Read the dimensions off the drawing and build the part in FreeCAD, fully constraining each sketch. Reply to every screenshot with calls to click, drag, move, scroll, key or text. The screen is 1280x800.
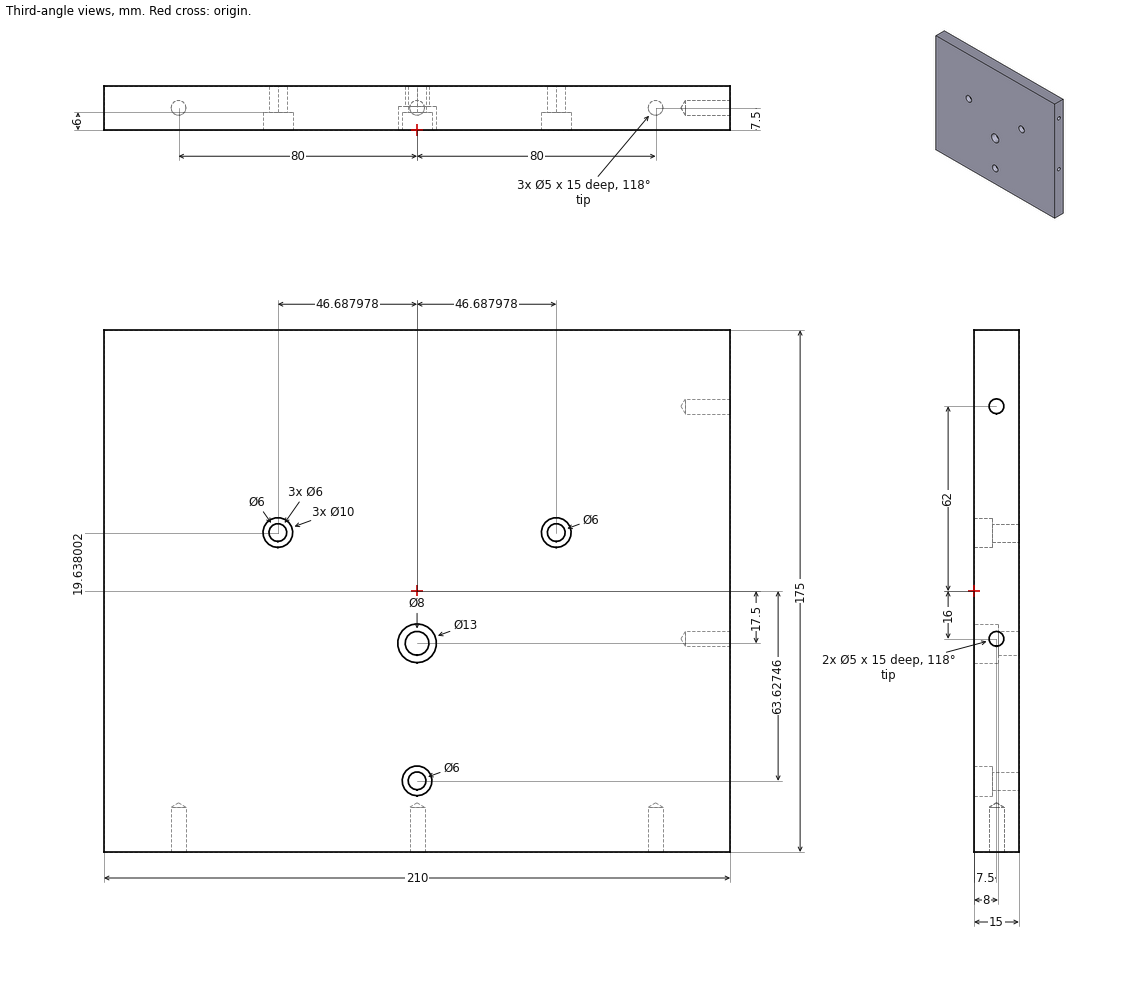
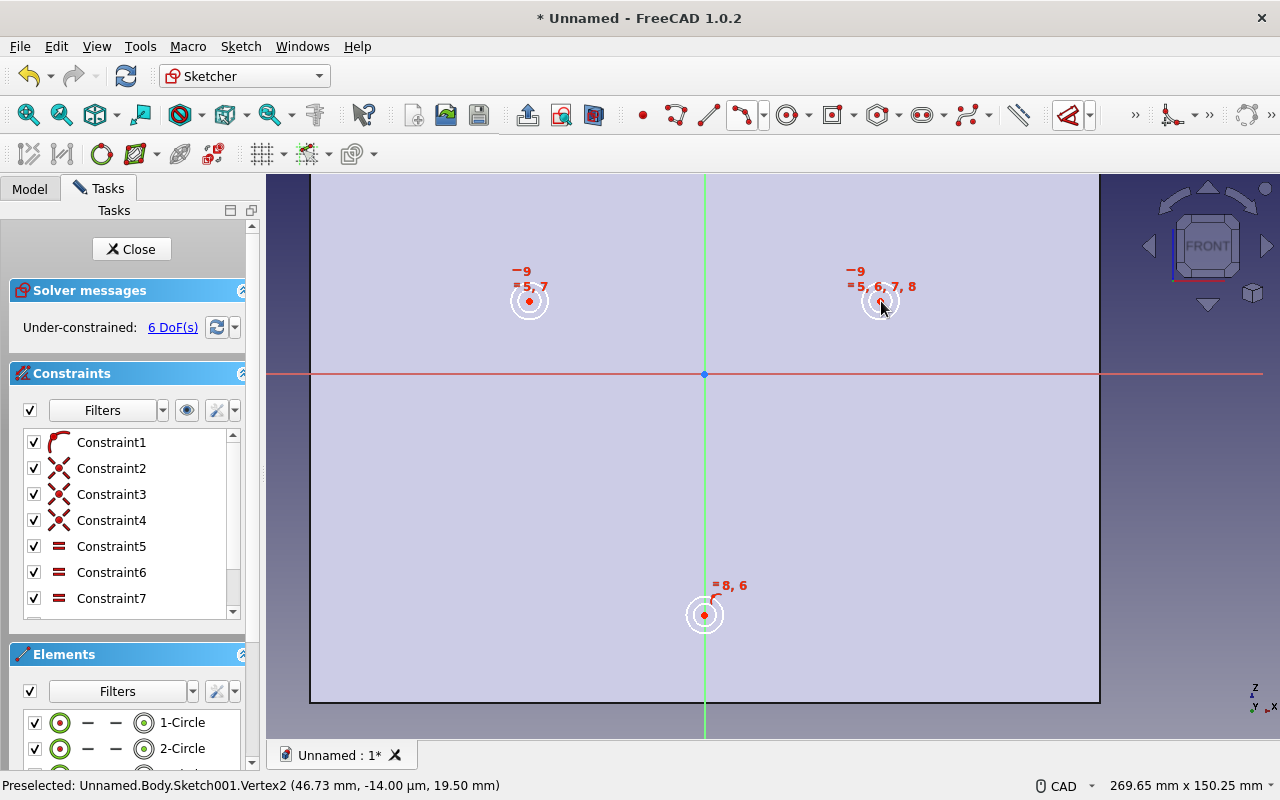
scroll(543, 288, up, 4)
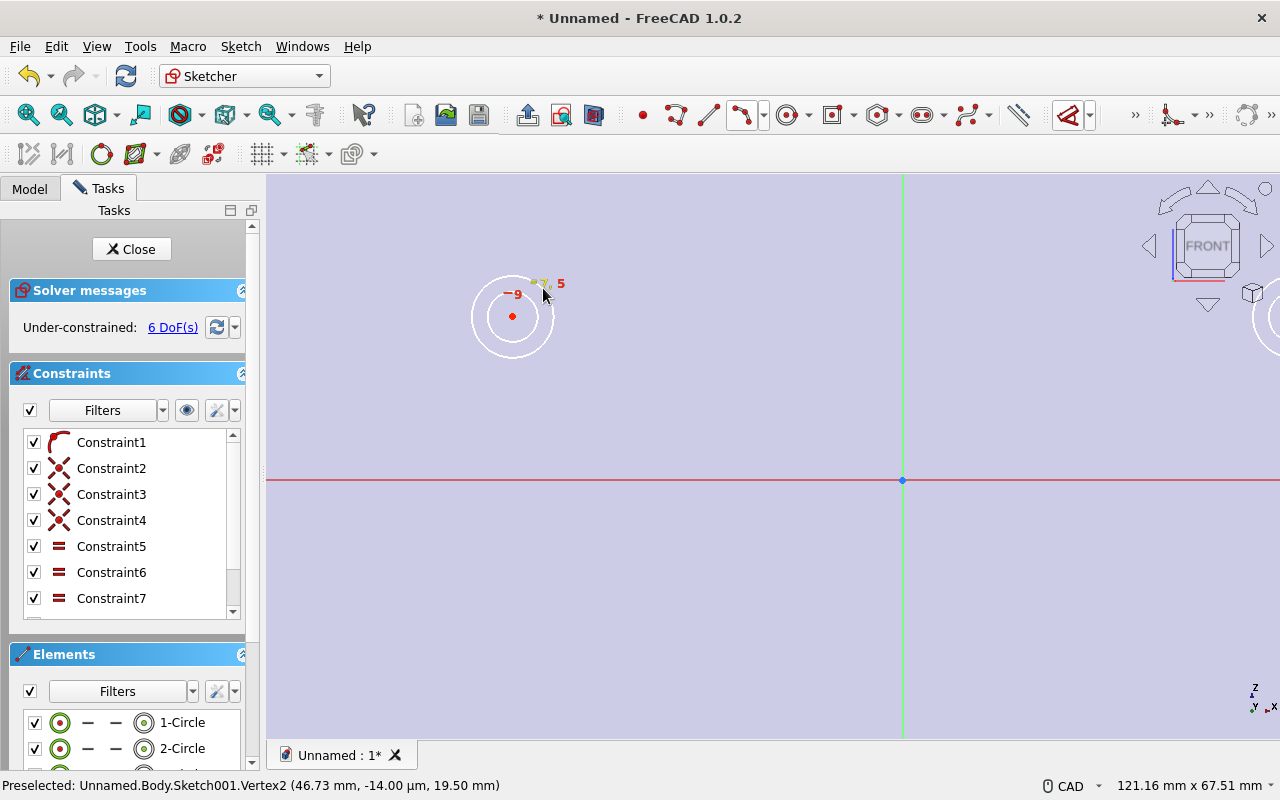
click(484, 346)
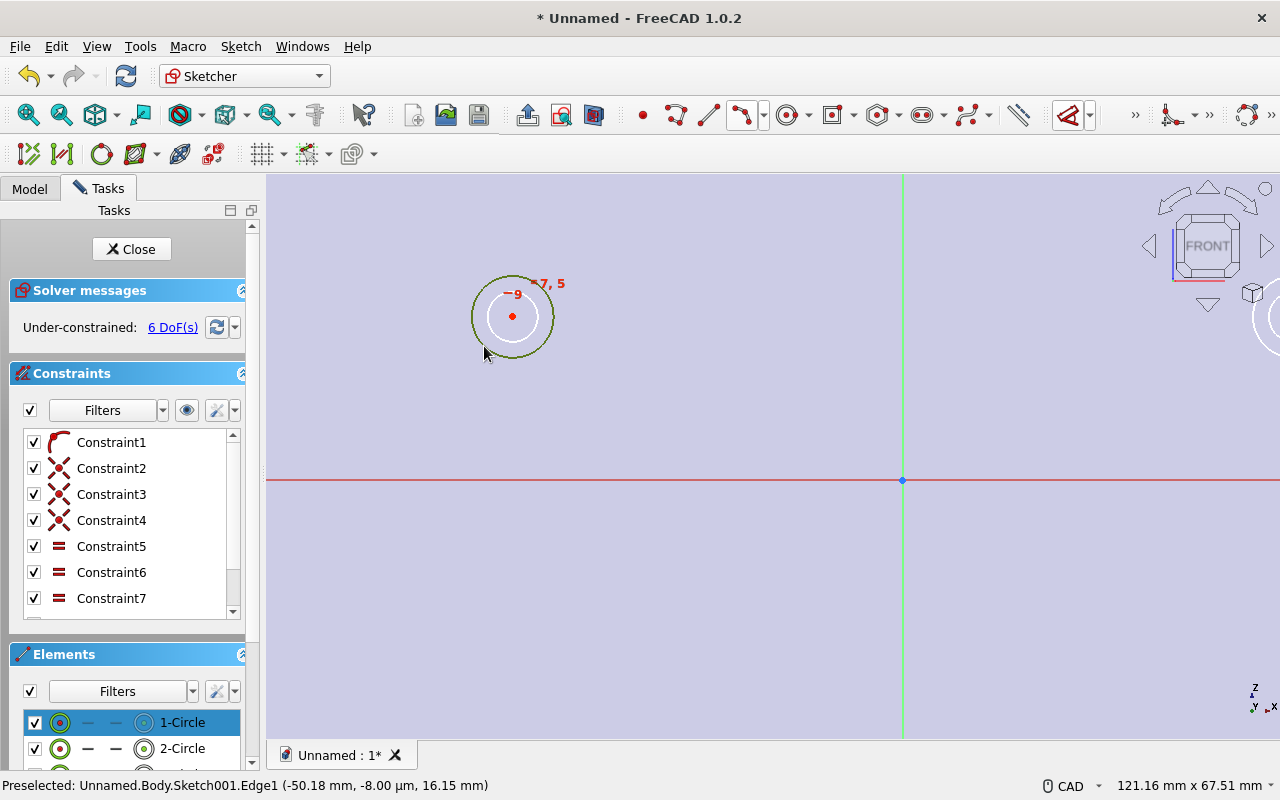
key(k)
key(o)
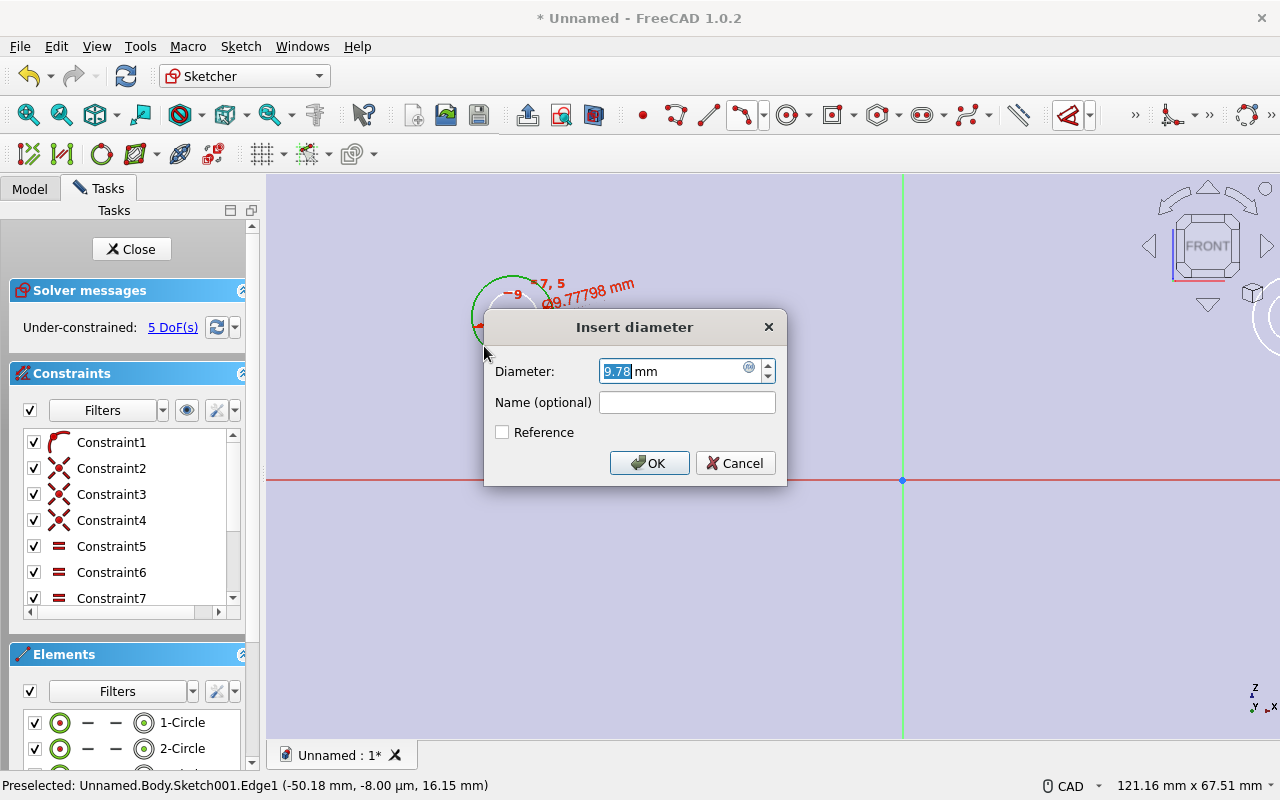
text(10)
key(Return)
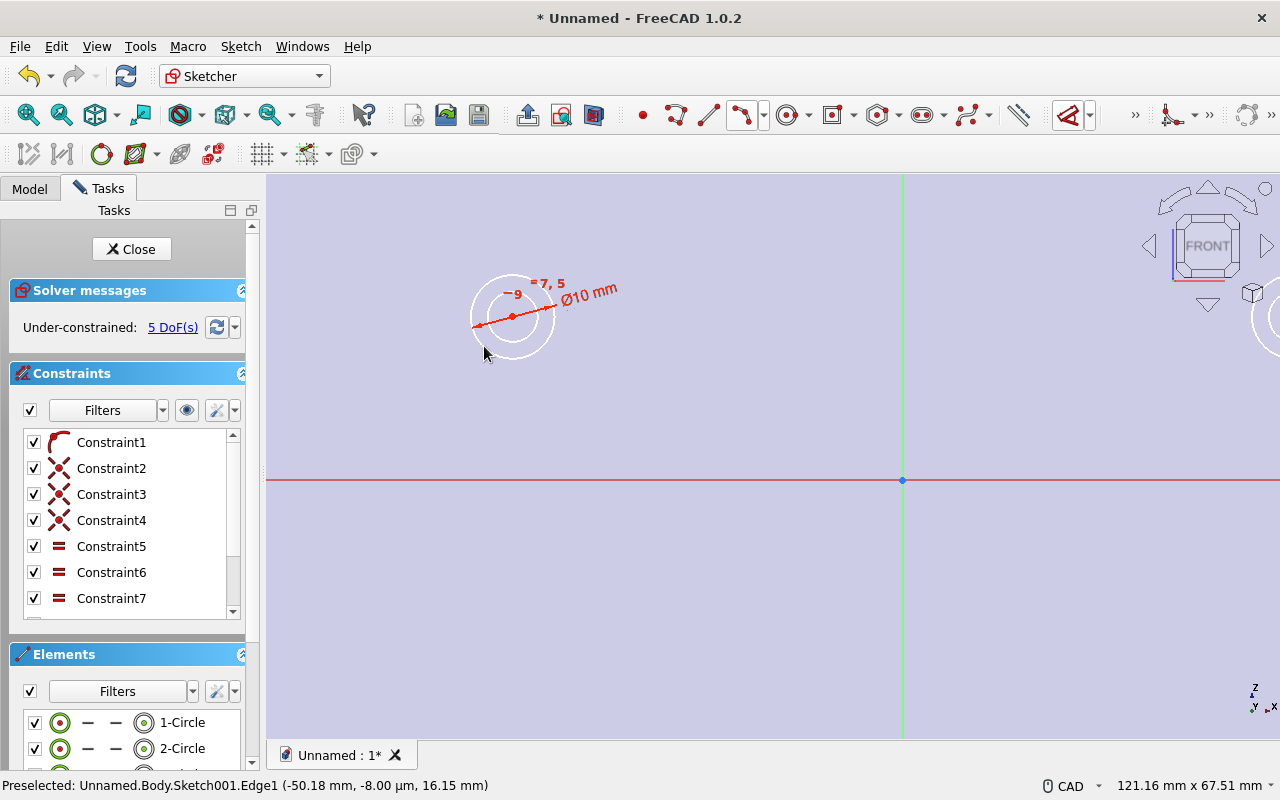
click(530, 299)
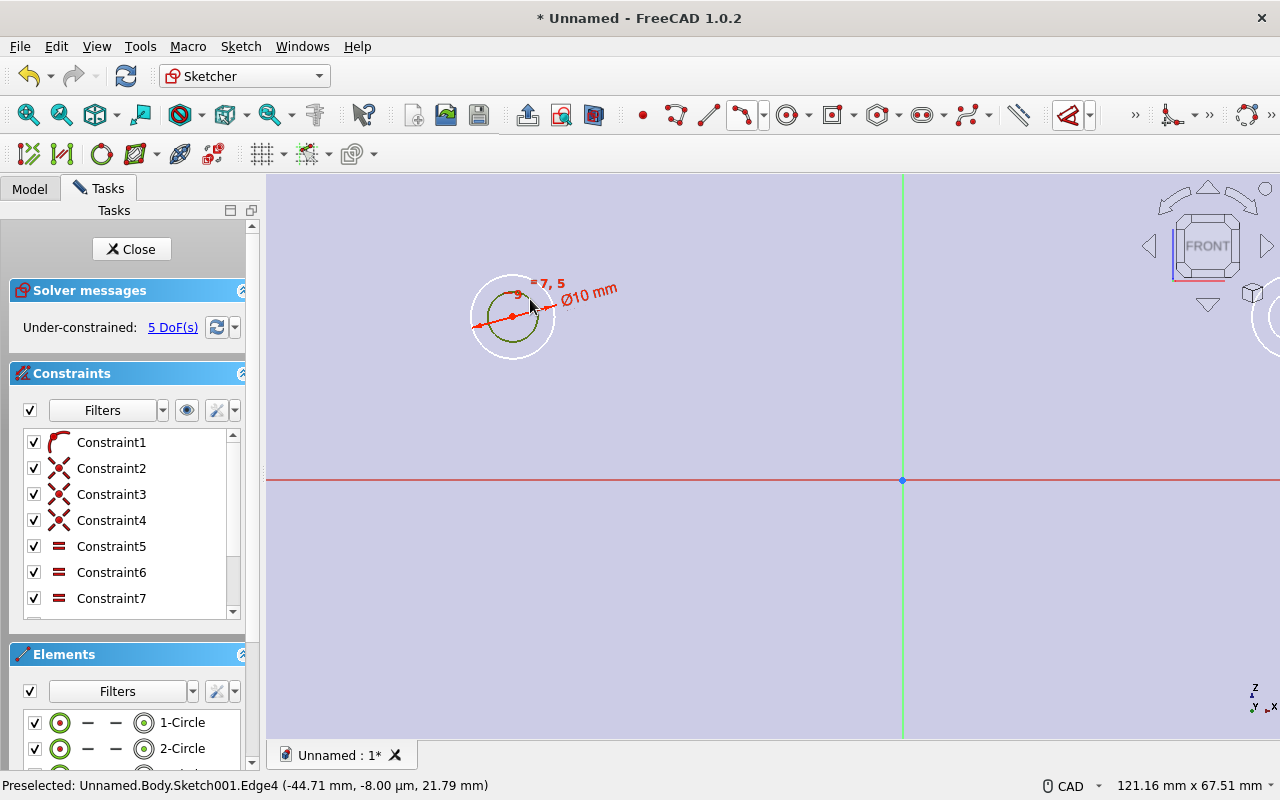
click(1090, 116)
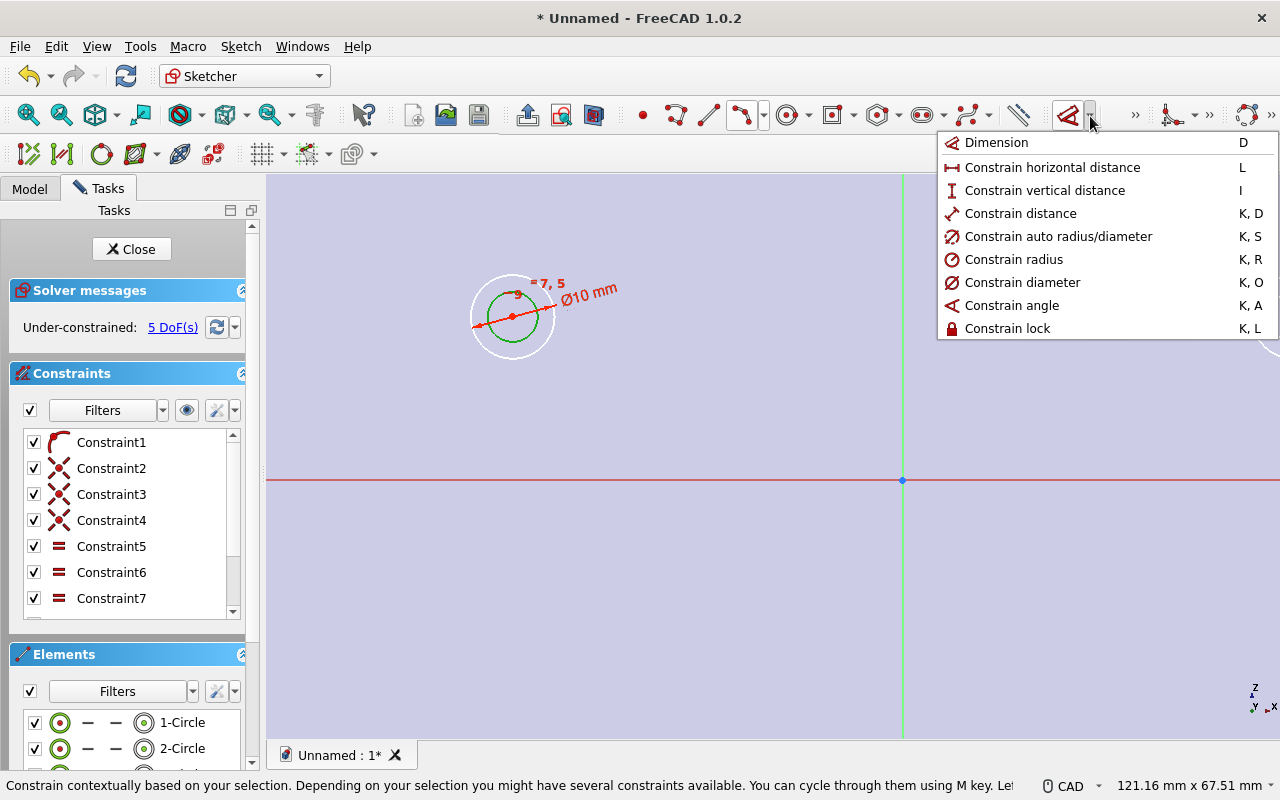
click(1108, 282)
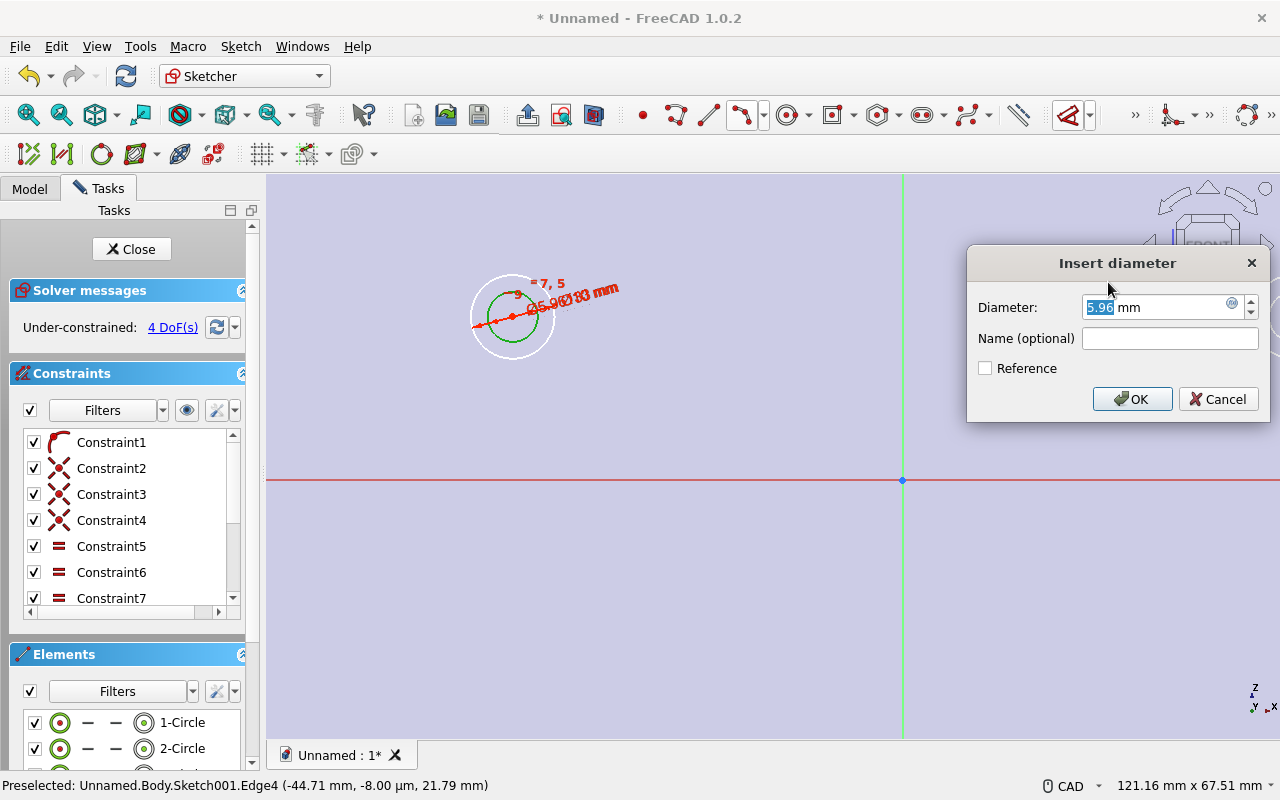
text(6)
key(Return)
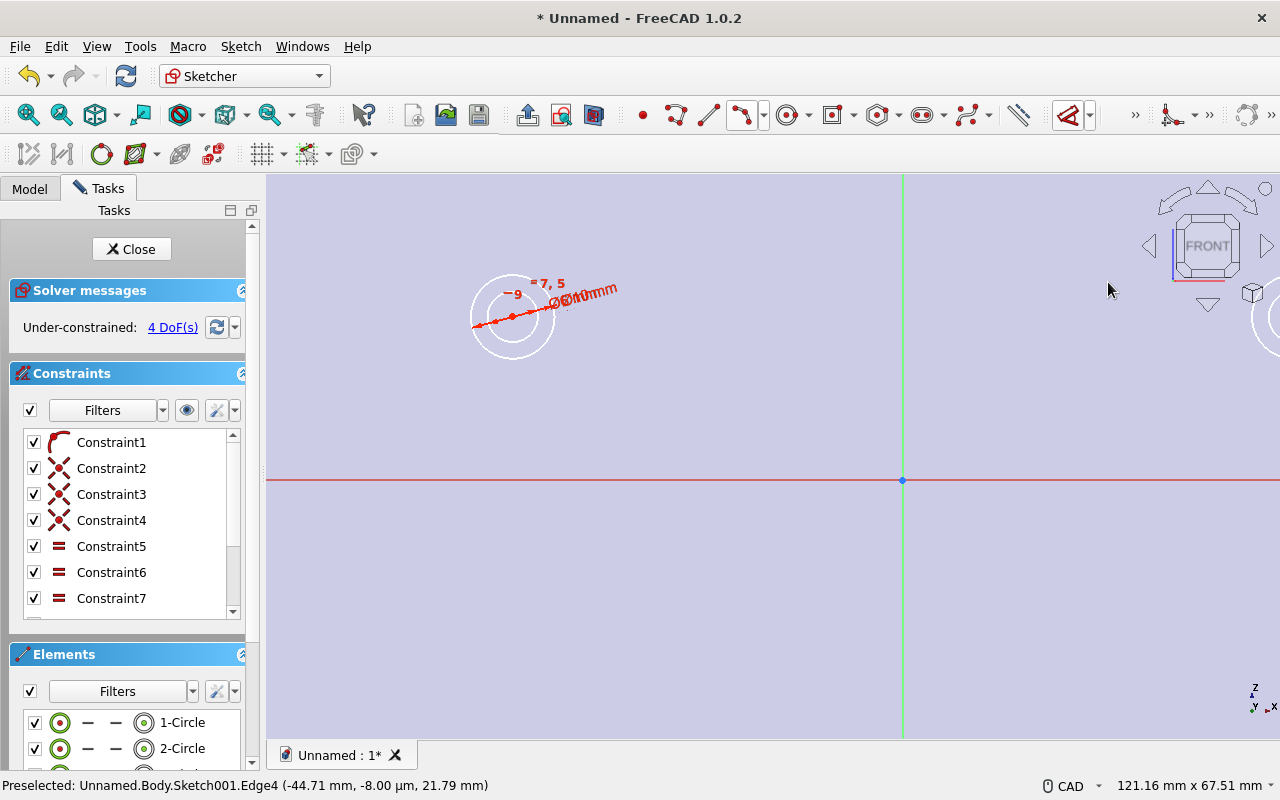
scroll(543, 287, down, 4)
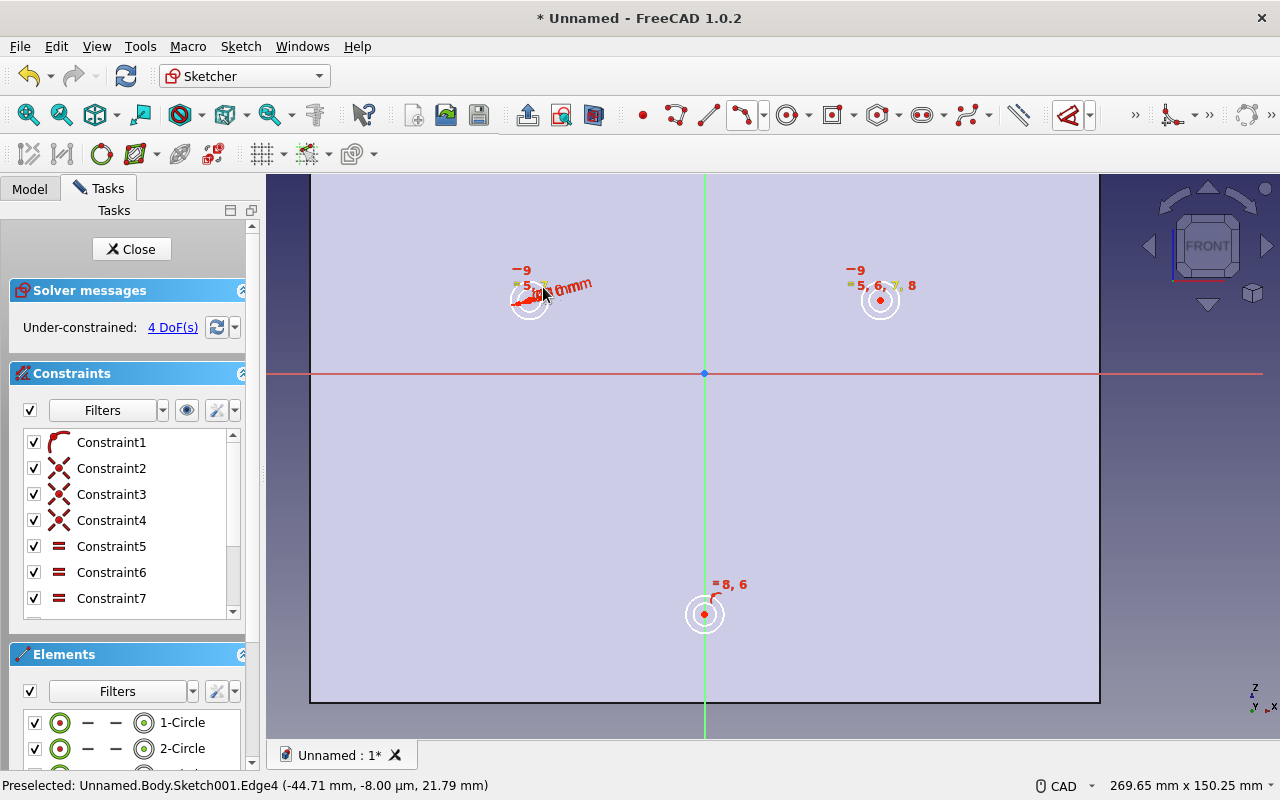
click(705, 615)